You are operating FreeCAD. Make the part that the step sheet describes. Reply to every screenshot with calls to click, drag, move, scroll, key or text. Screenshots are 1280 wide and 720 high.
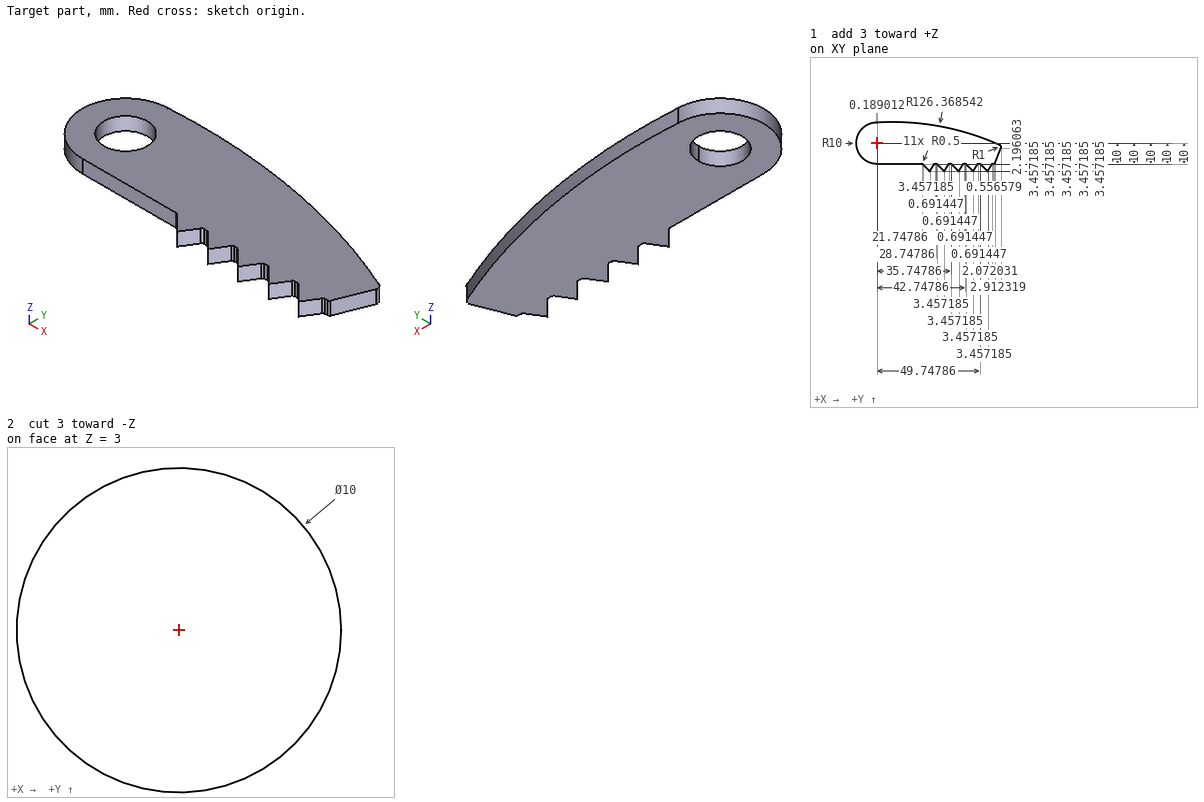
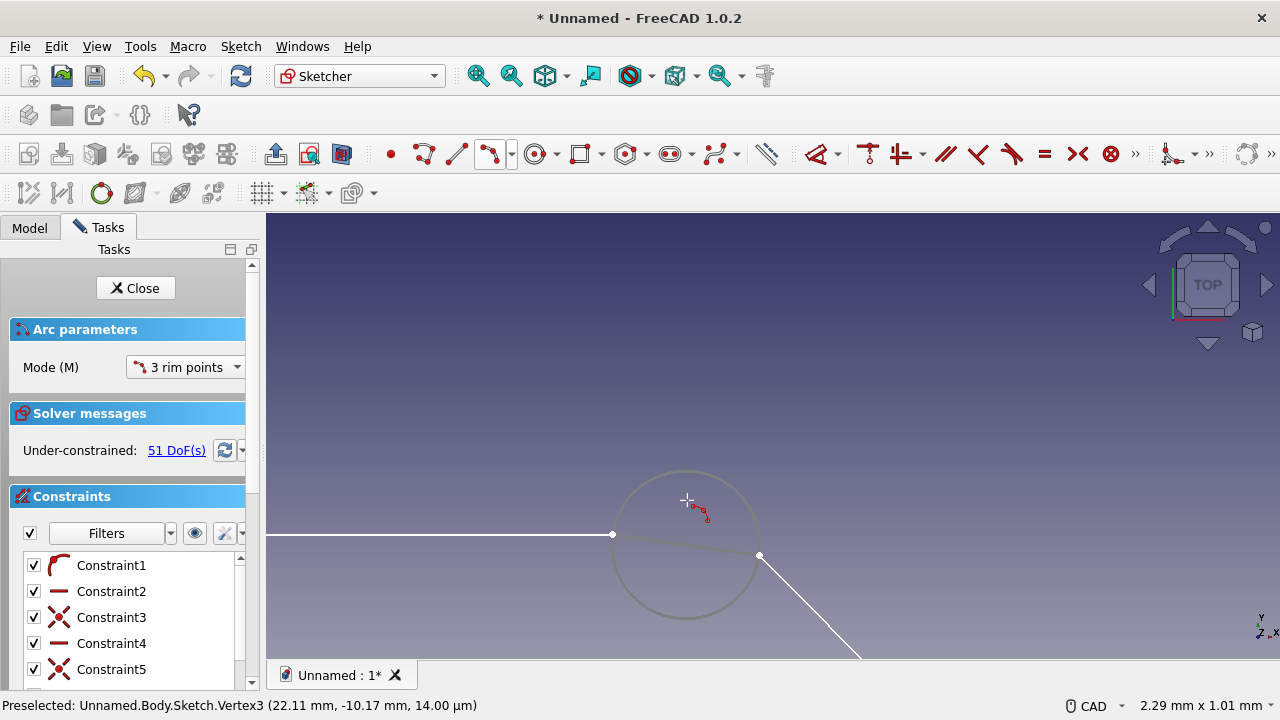
click(684, 498)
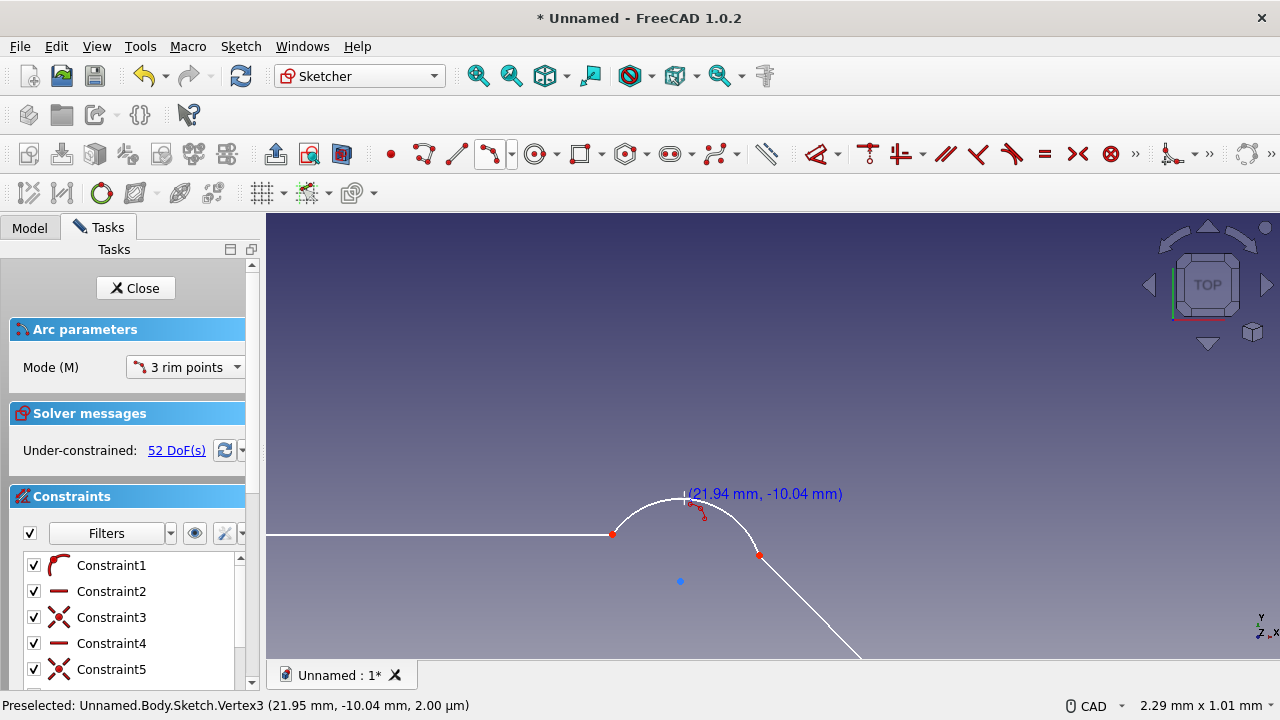
scroll(704, 436, down, 15)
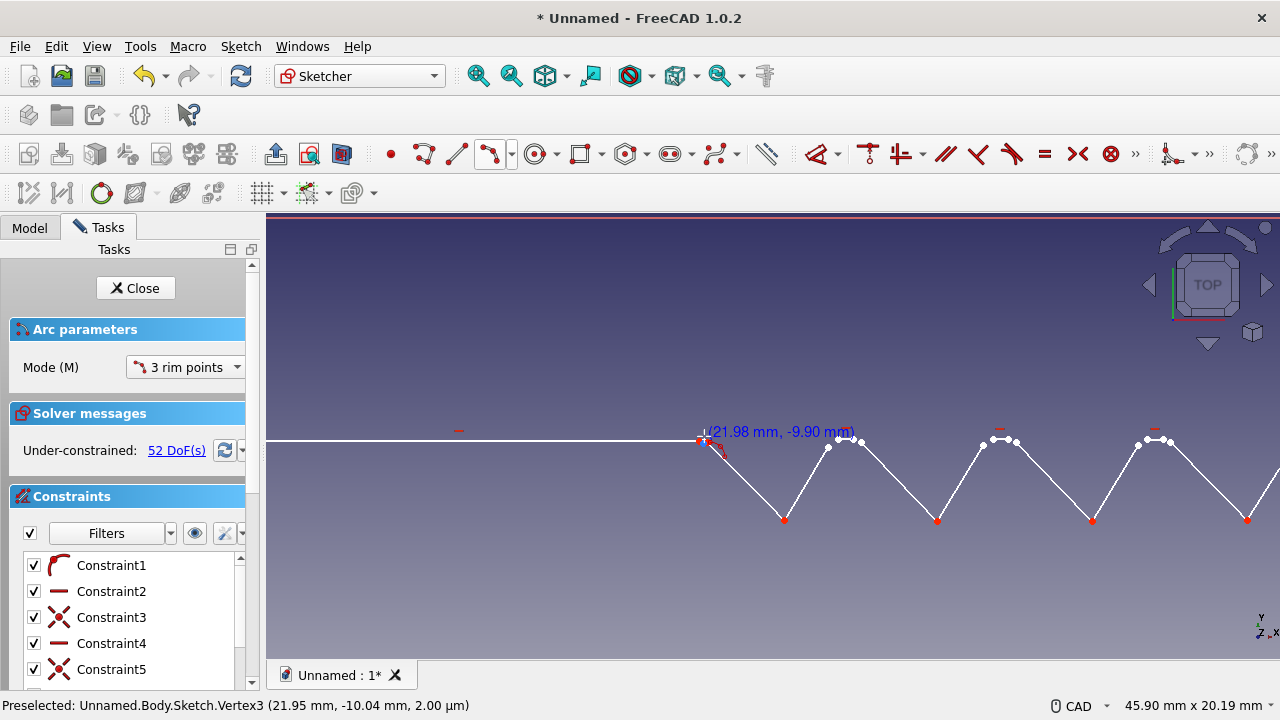
scroll(666, 540, down, 5)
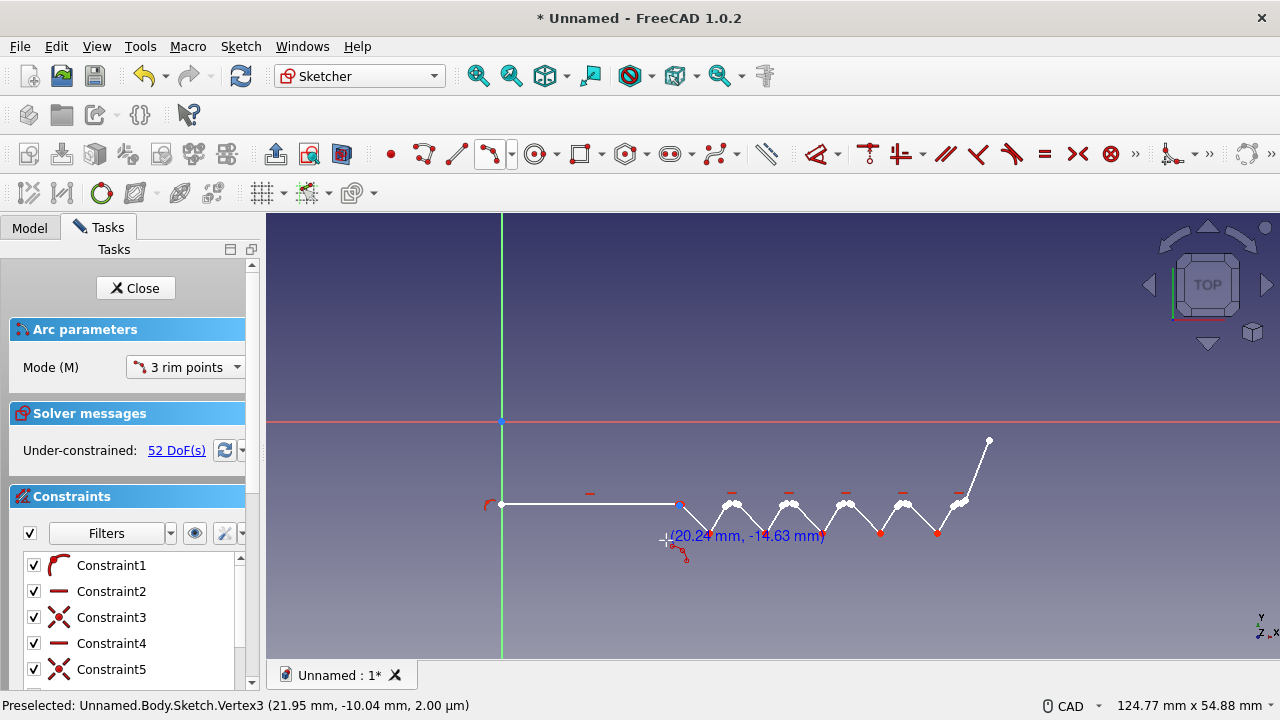
scroll(726, 505, up, 7)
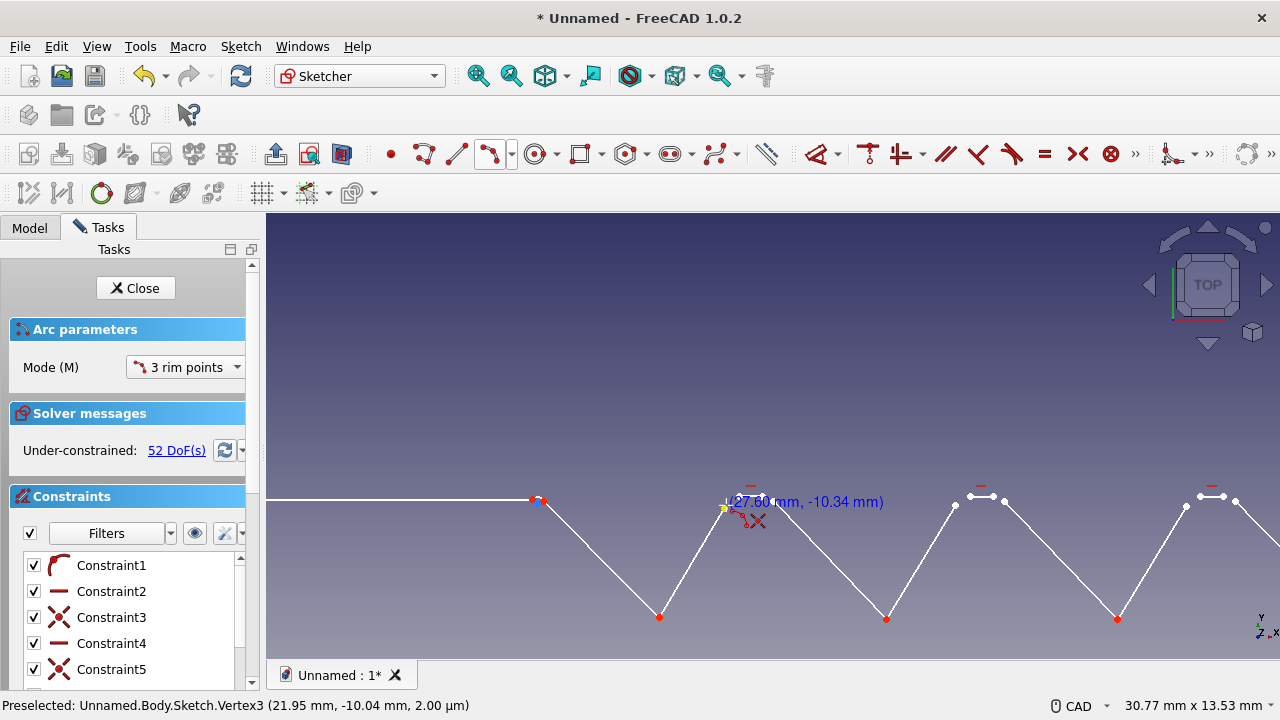
click(724, 508)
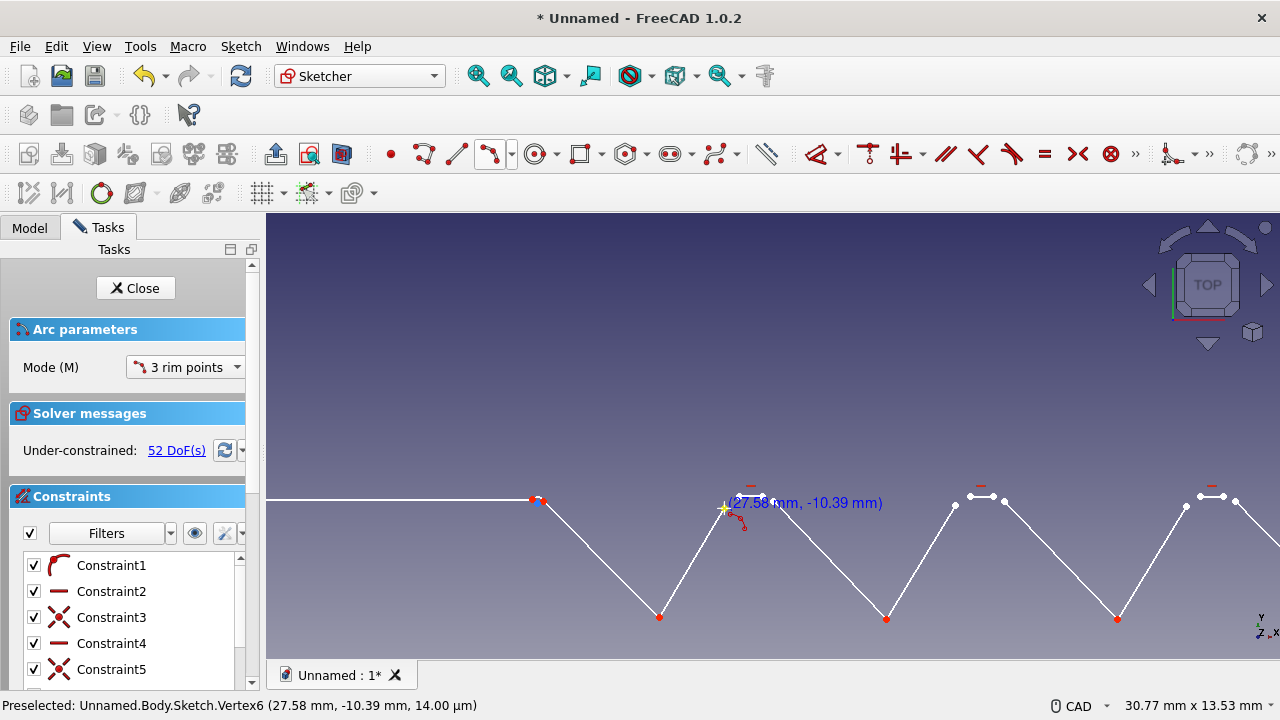
scroll(740, 496, up, 2)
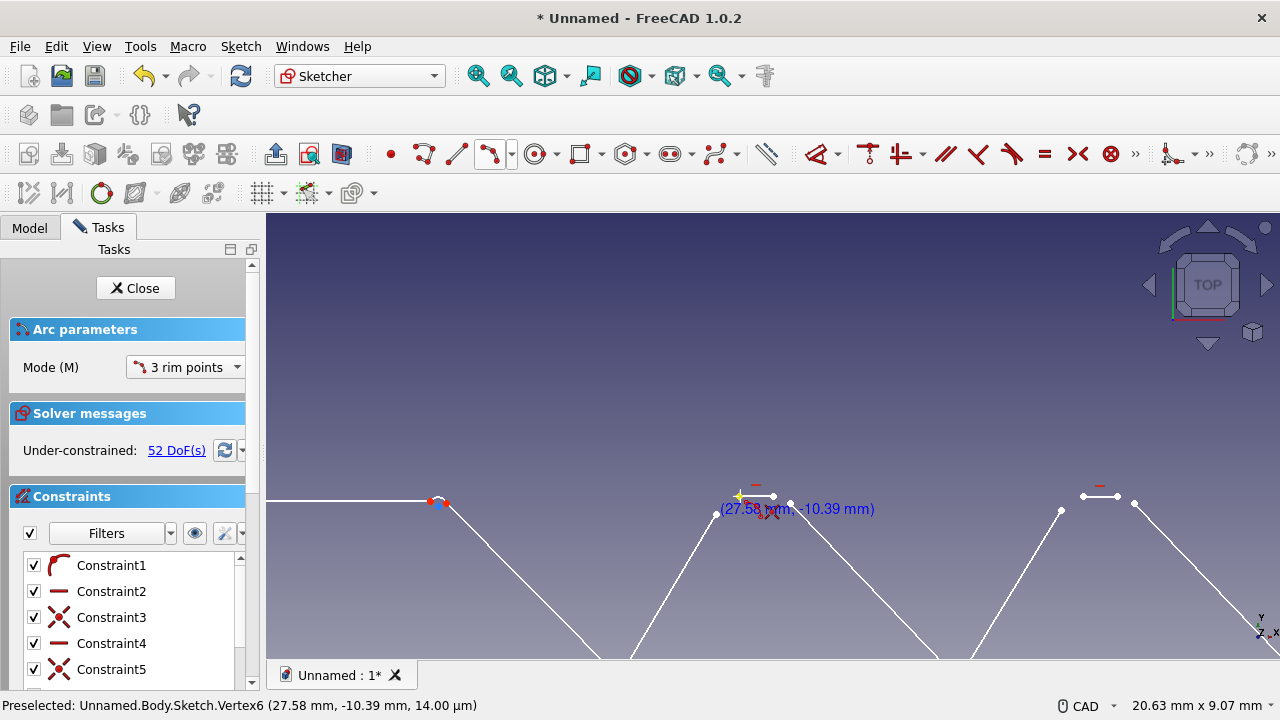
click(739, 496)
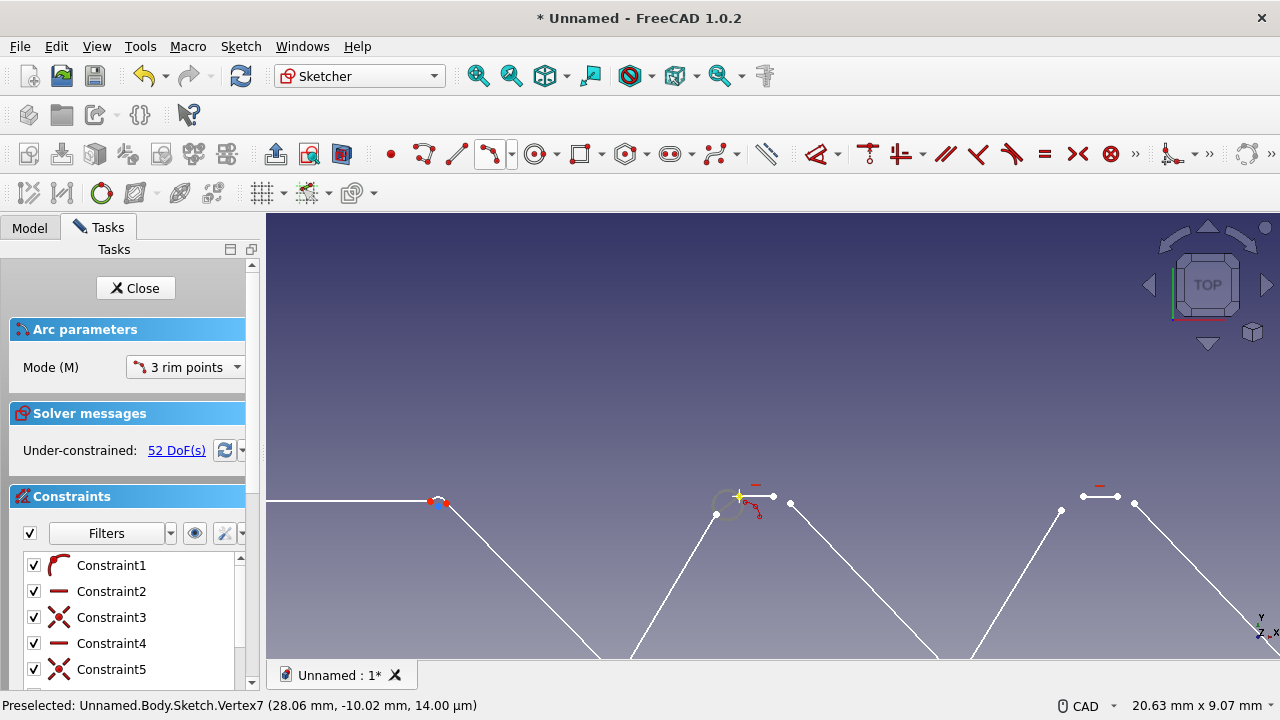
scroll(727, 498, up, 9)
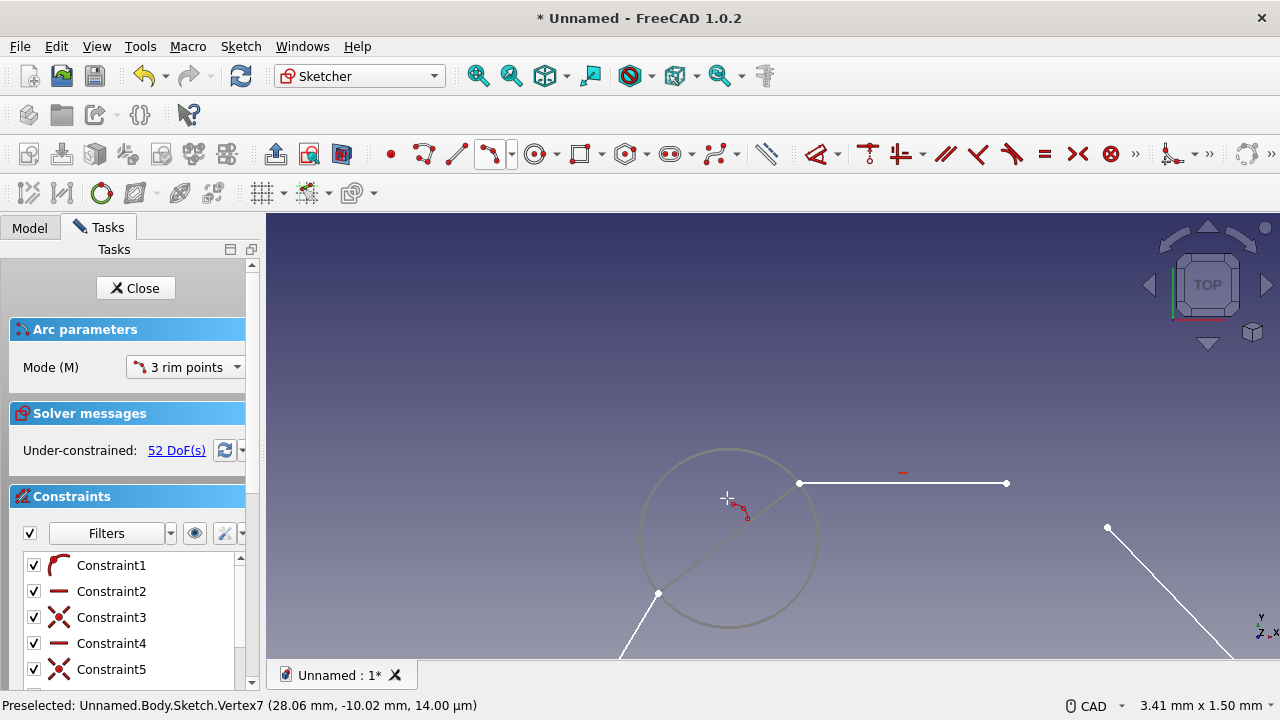
click(727, 497)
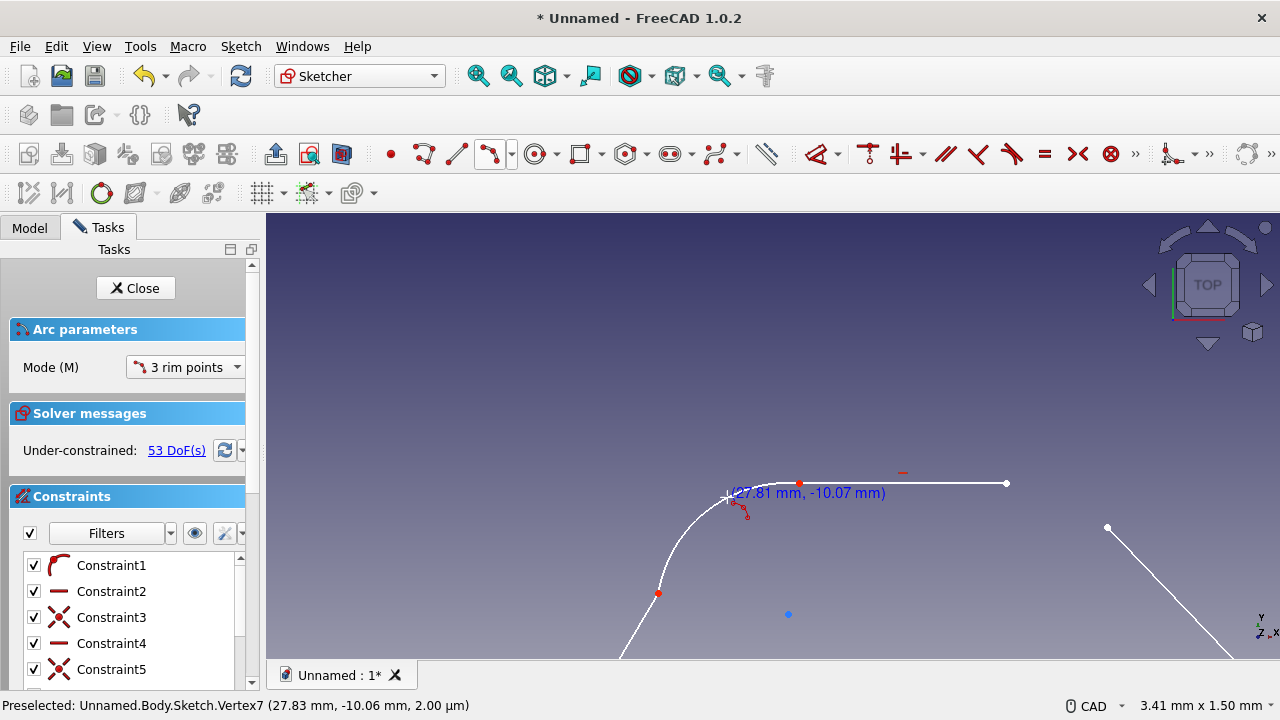
scroll(733, 519, down, 17)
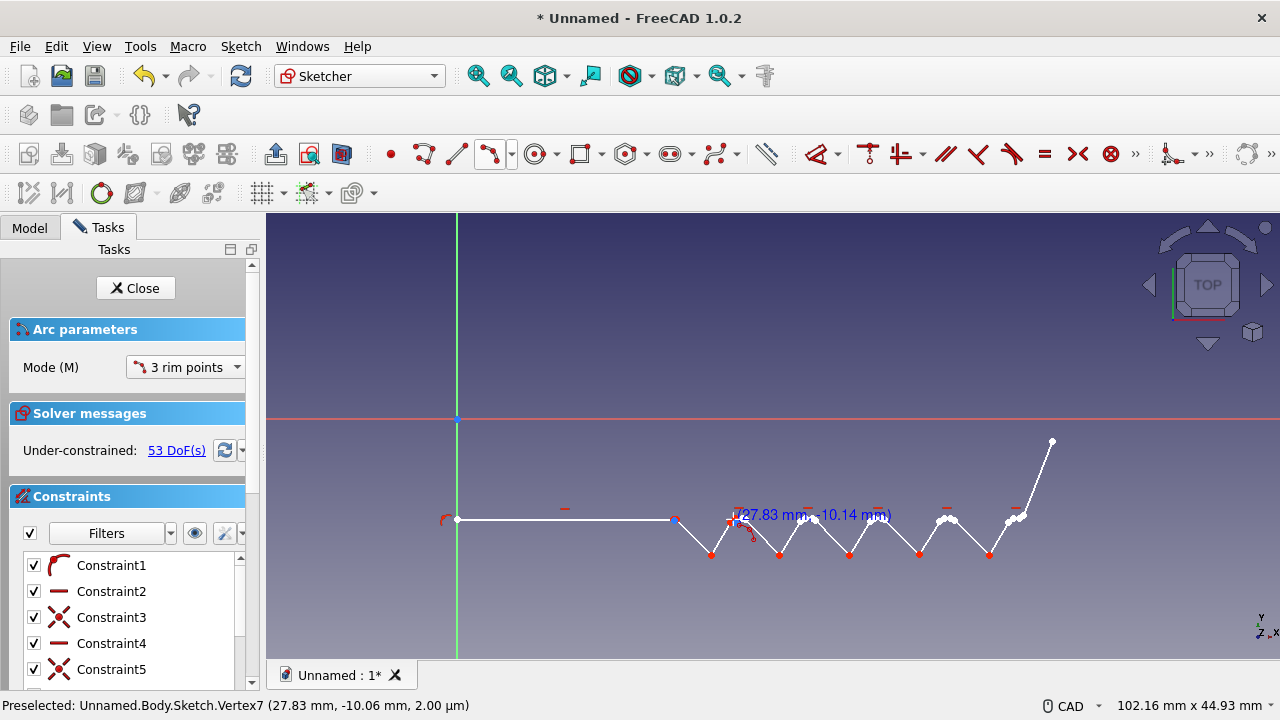
scroll(743, 518, up, 8)